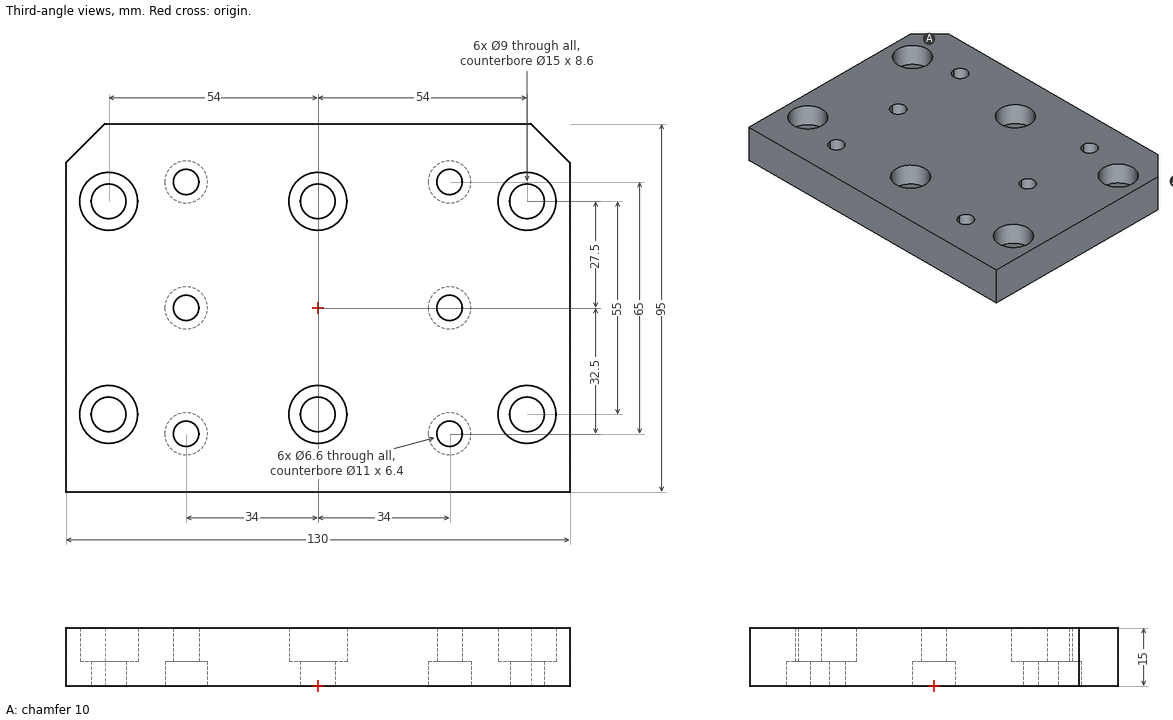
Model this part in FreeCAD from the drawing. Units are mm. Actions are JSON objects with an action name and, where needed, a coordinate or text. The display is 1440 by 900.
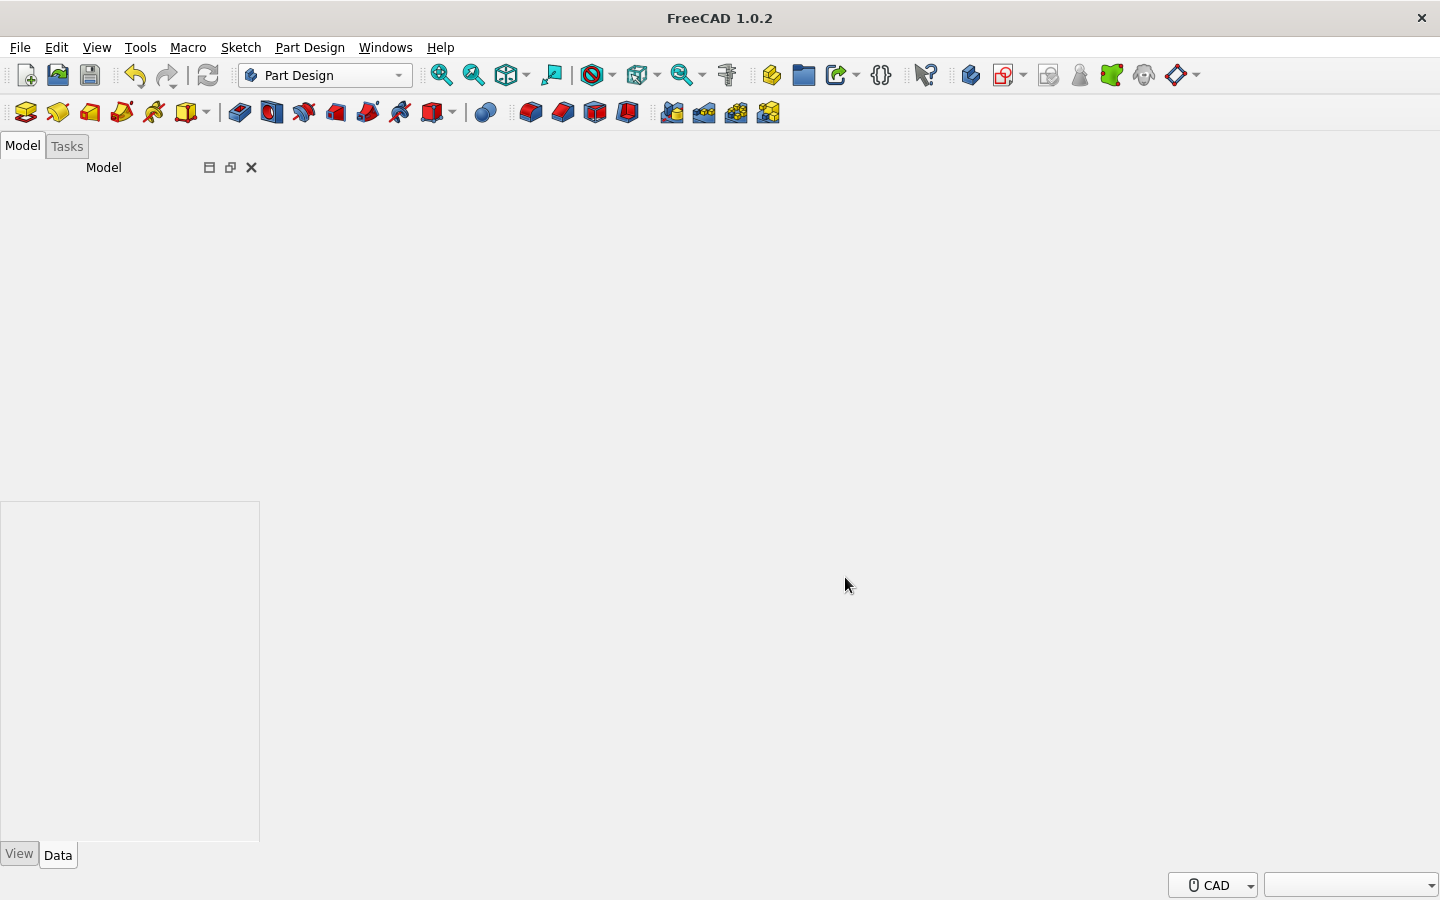
{"action": "key", "text": "ctrl+n"}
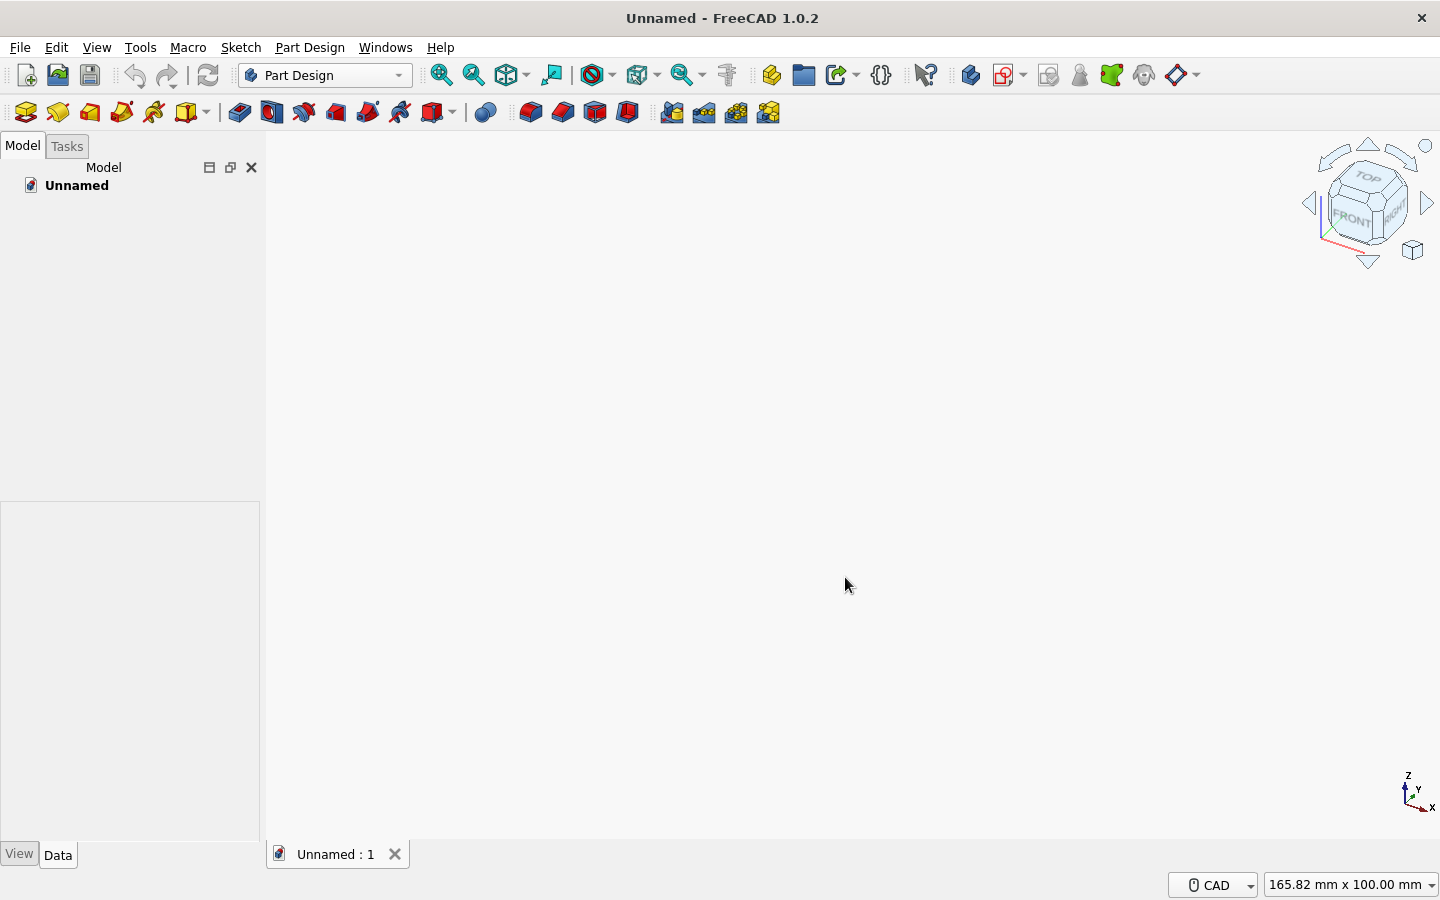
{"action": "left_click", "coordinate": [1004, 76]}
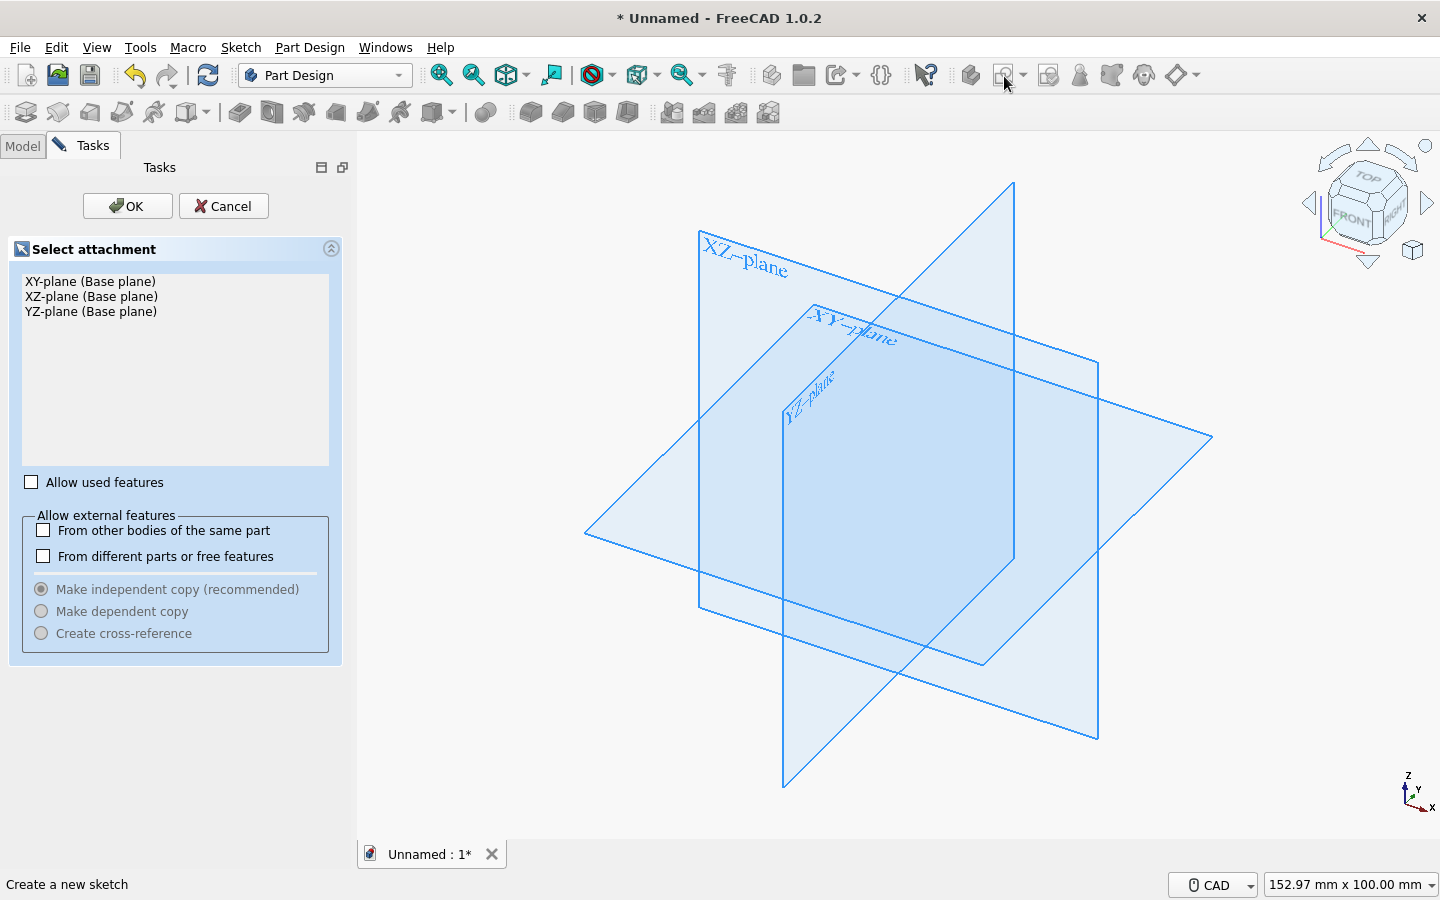
{"action": "left_click", "coordinate": [82, 282]}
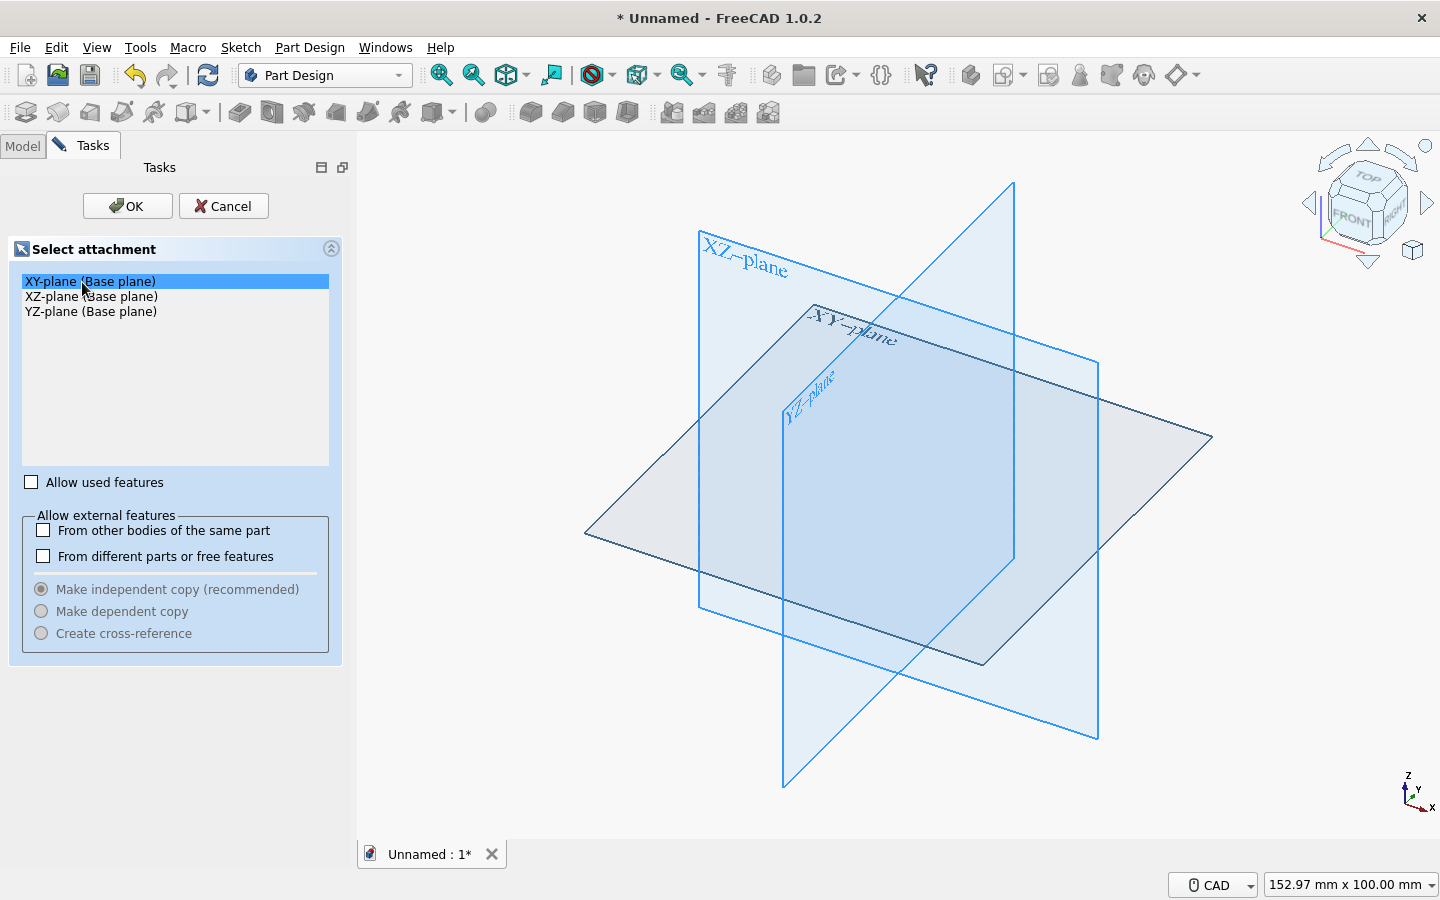
{"action": "left_click", "coordinate": [128, 206]}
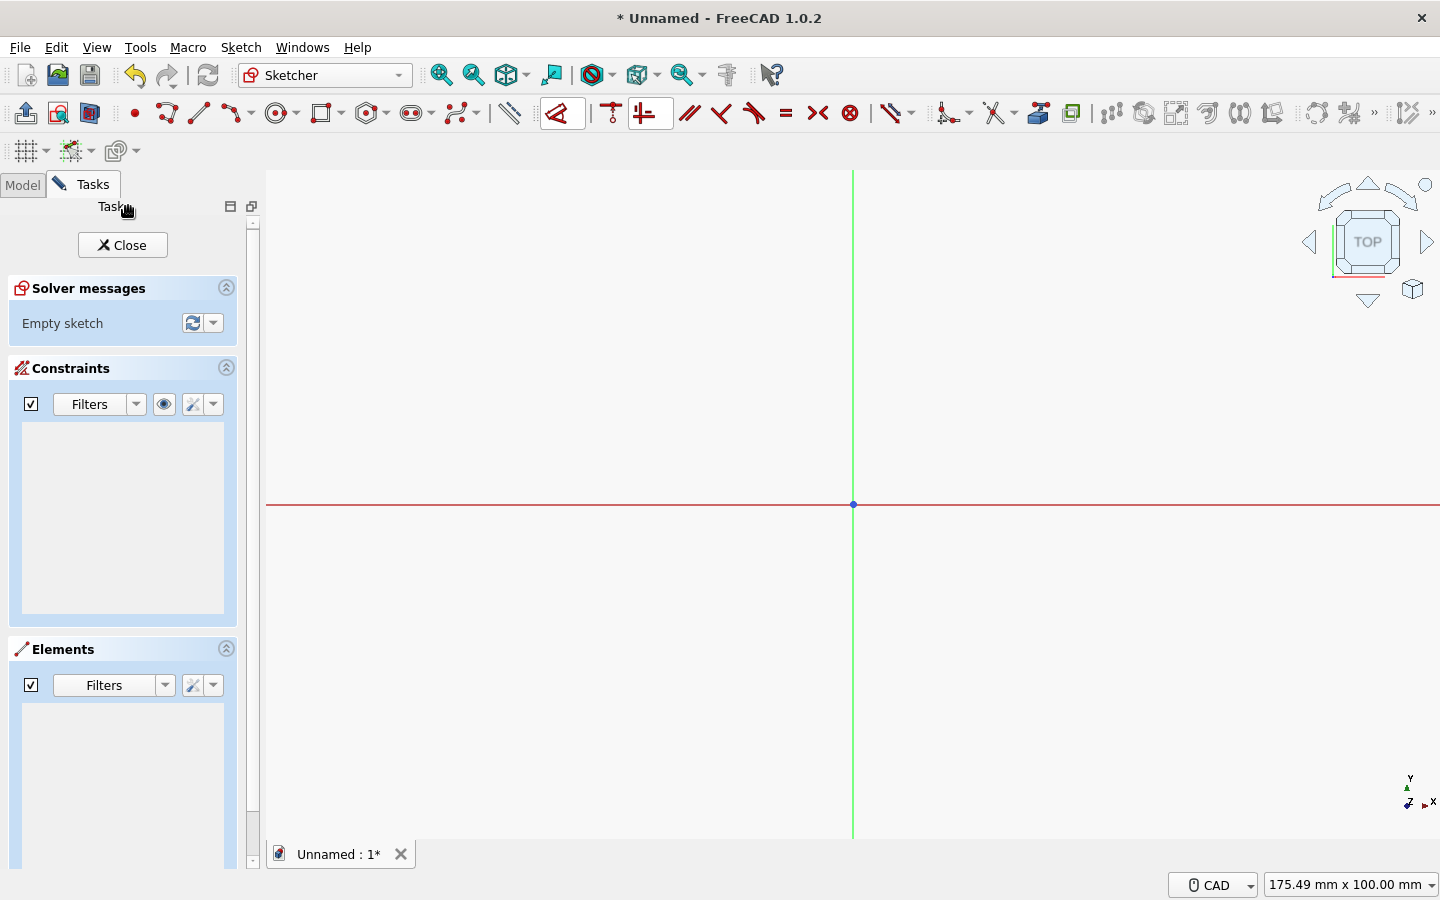
{"action": "scroll", "coordinate": [645, 504], "scroll_direction": "down", "scroll_amount": 2}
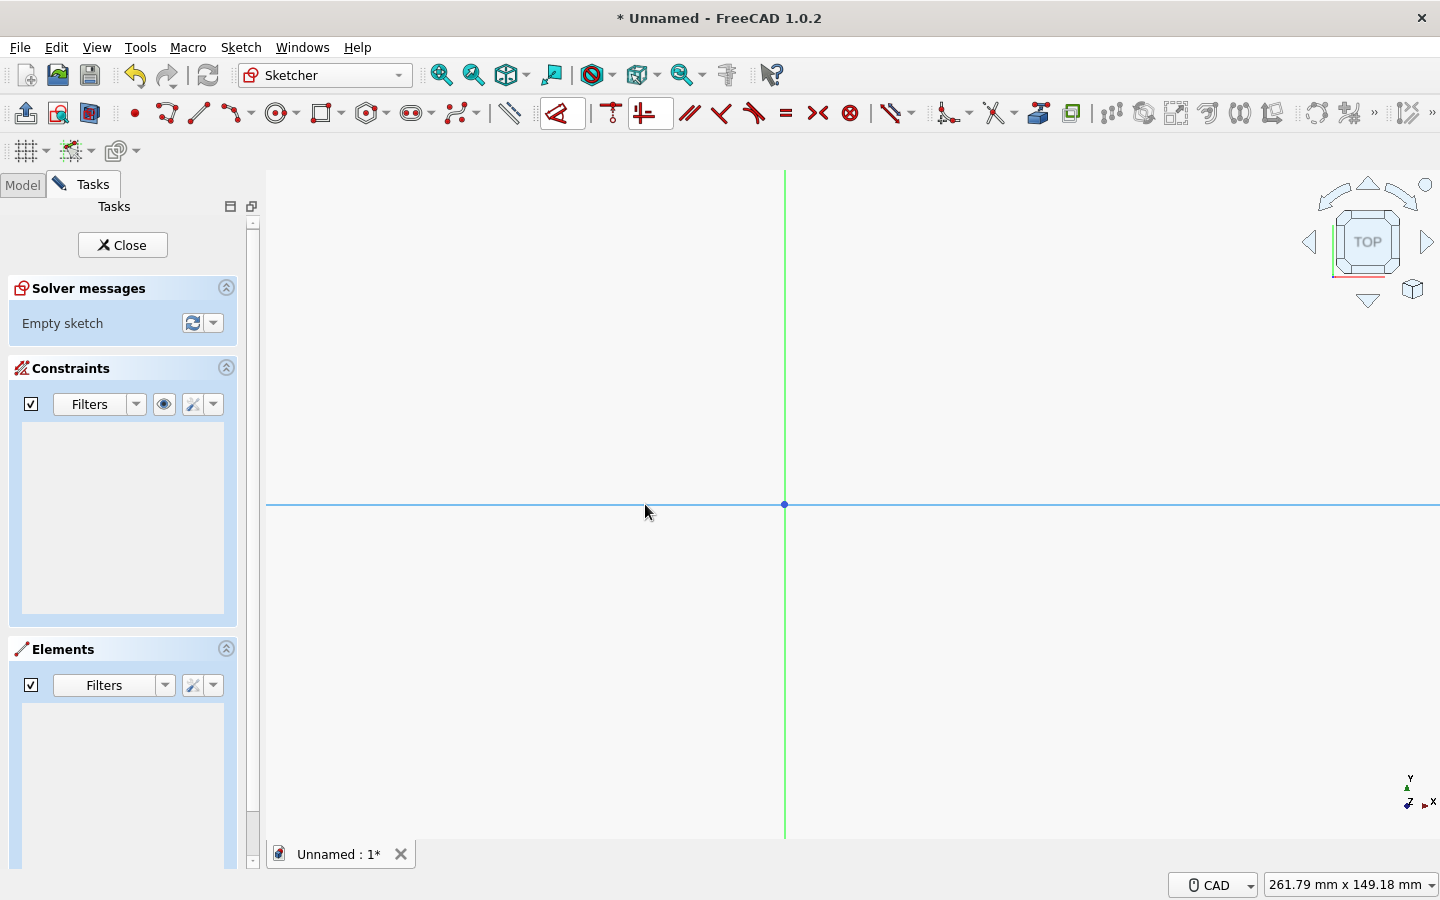
{"action": "key", "text": "g v"}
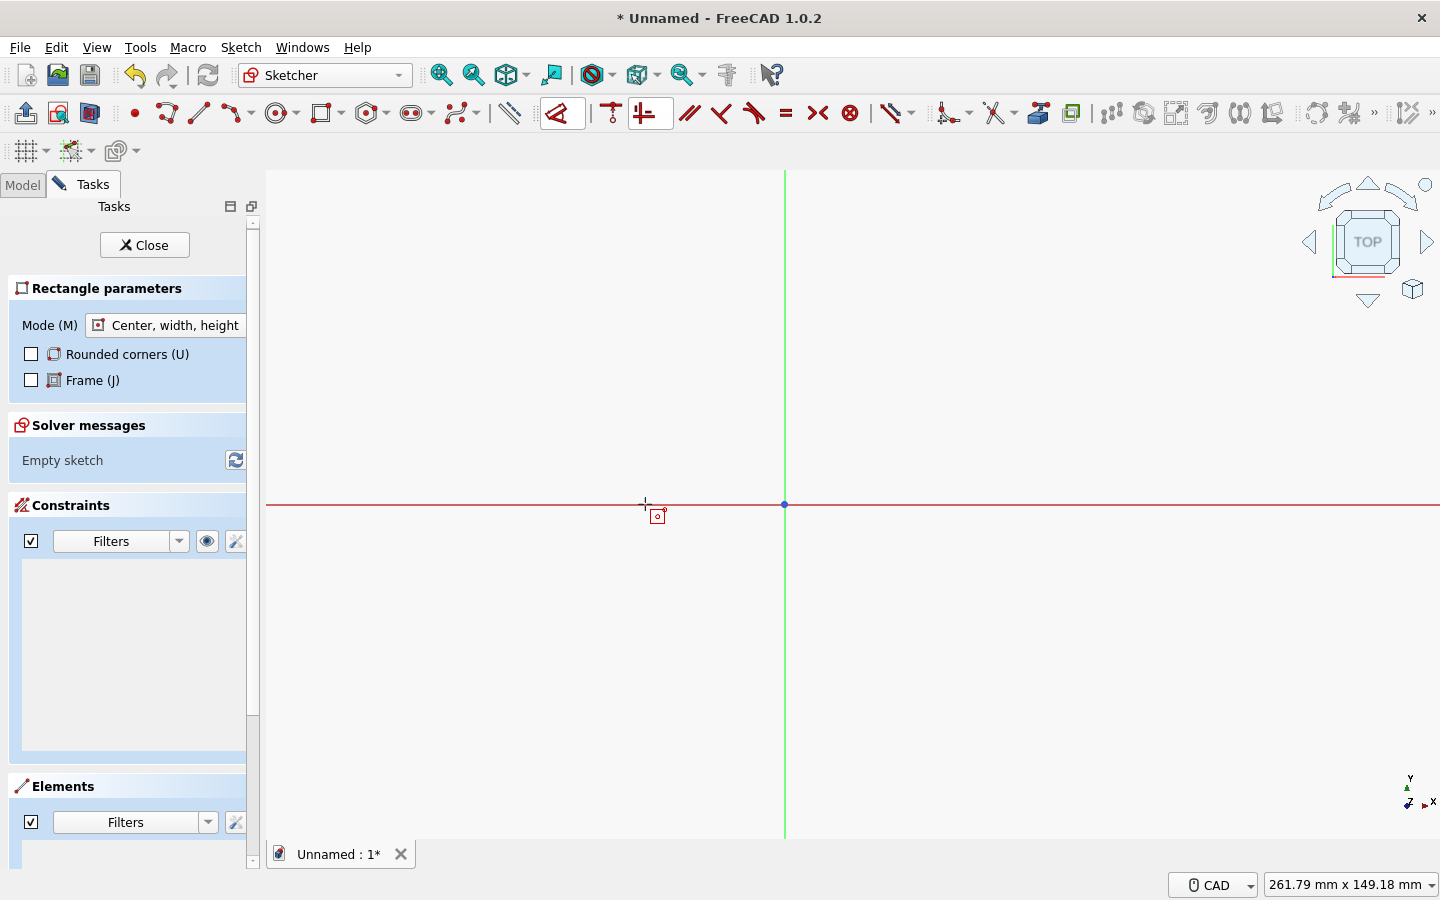
{"action": "left_click", "coordinate": [785, 504]}
{"action": "mouse_move", "coordinate": [1076, 291]}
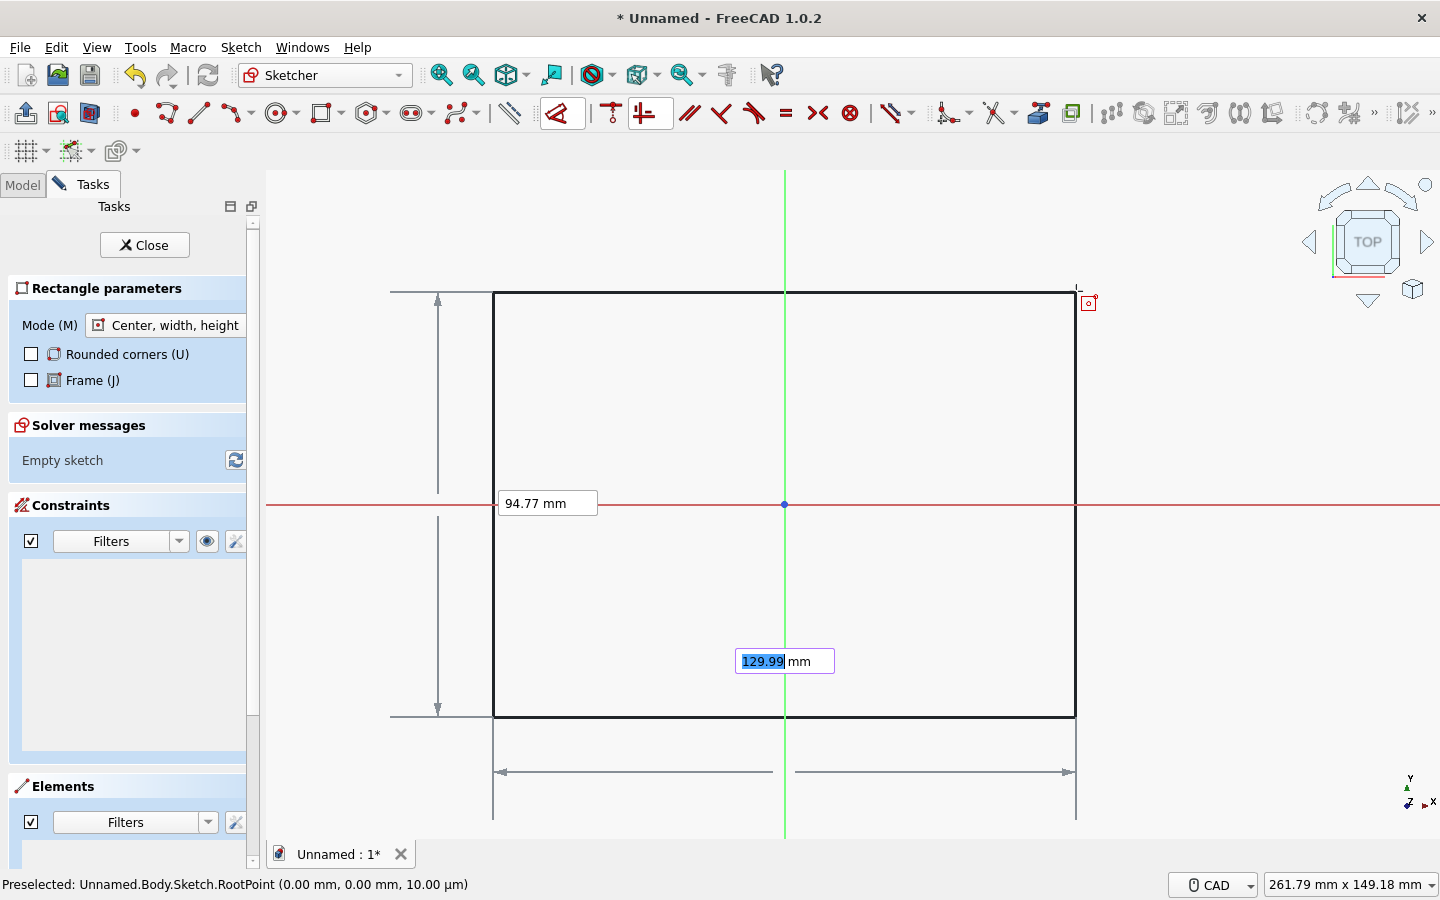
{"action": "type", "text": "130"}
{"action": "key", "text": "Tab"}
{"action": "type", "text": "95"}
{"action": "key", "text": "Return"}
{"action": "key", "text": "Escape"}